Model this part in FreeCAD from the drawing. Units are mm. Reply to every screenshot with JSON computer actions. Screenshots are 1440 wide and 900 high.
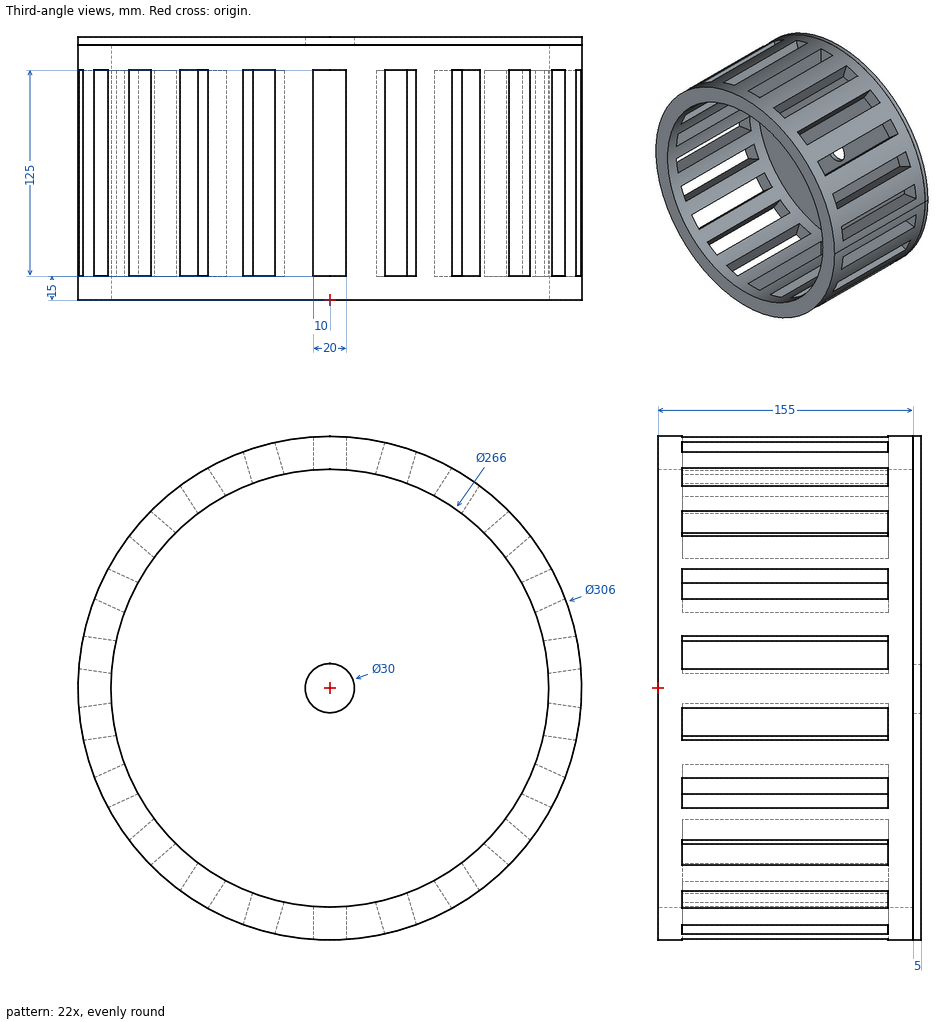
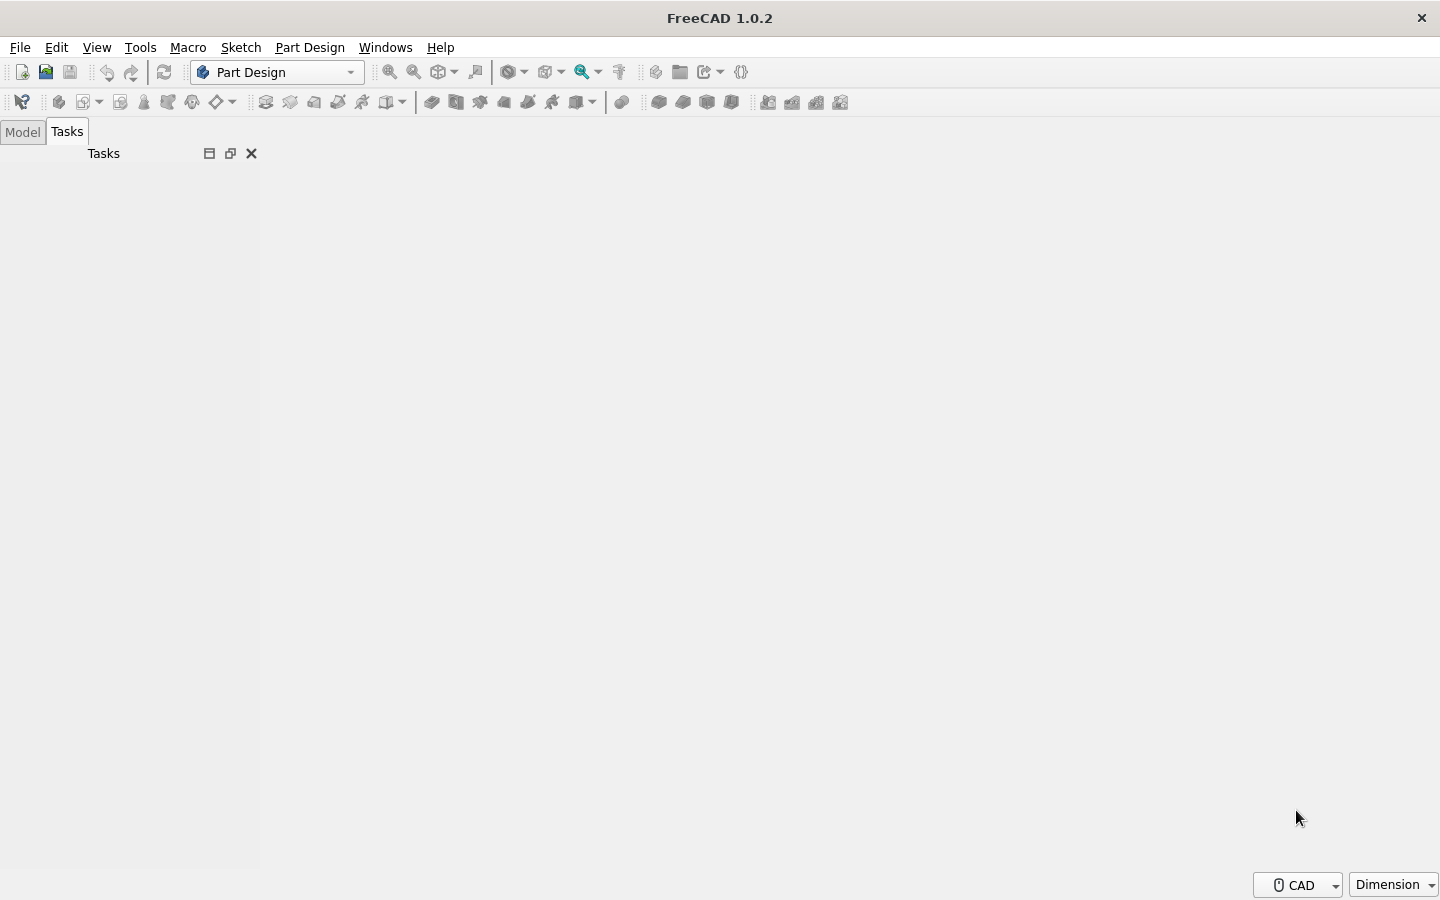
{"action": "left_click", "coordinate": [22, 72]}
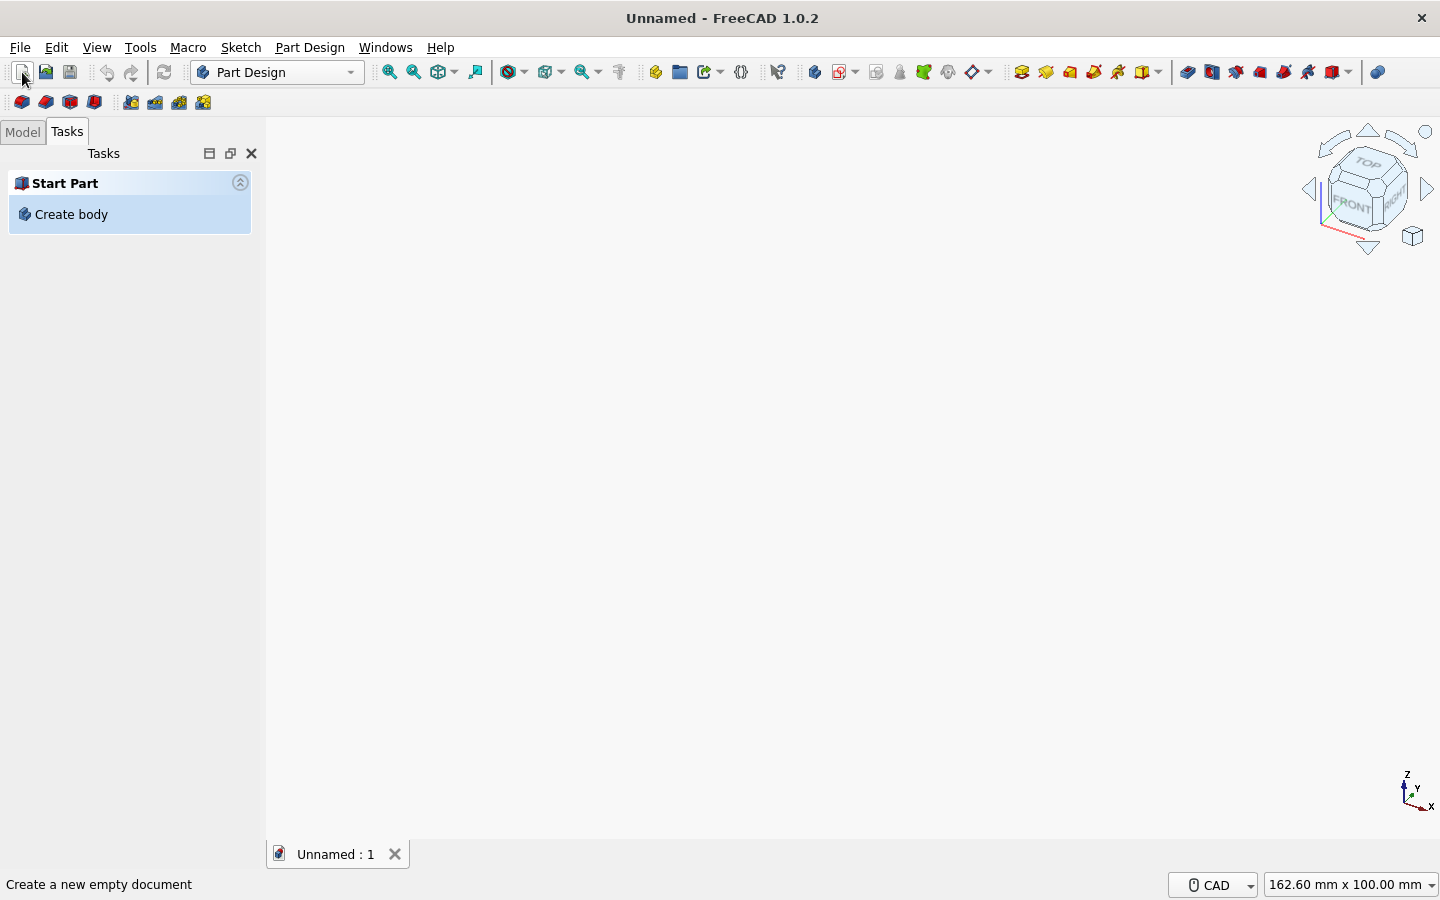
{"action": "left_click", "coordinate": [840, 72]}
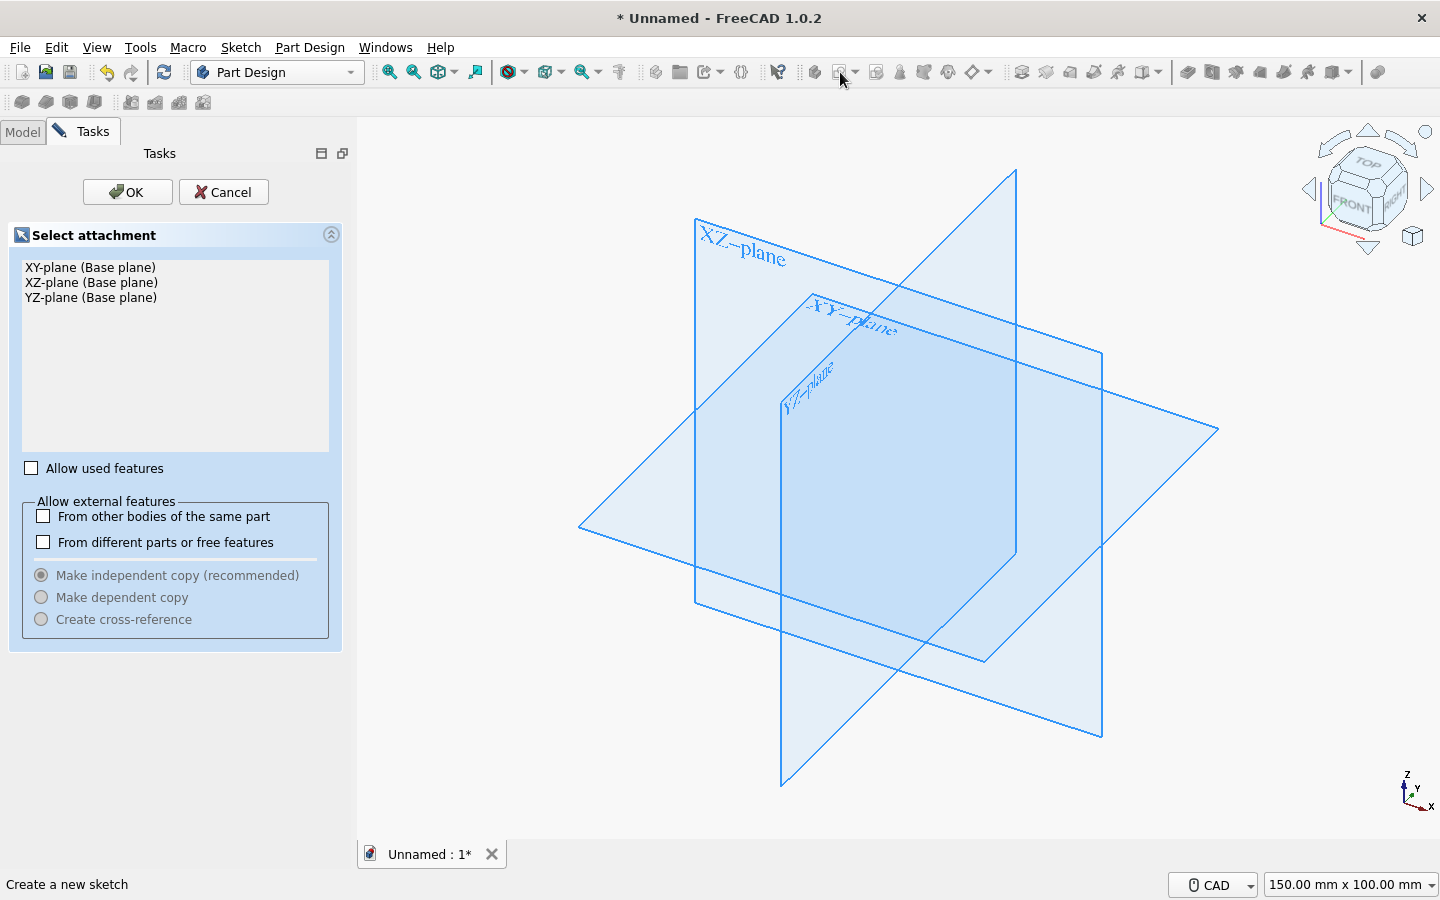
{"action": "left_click", "coordinate": [82, 282]}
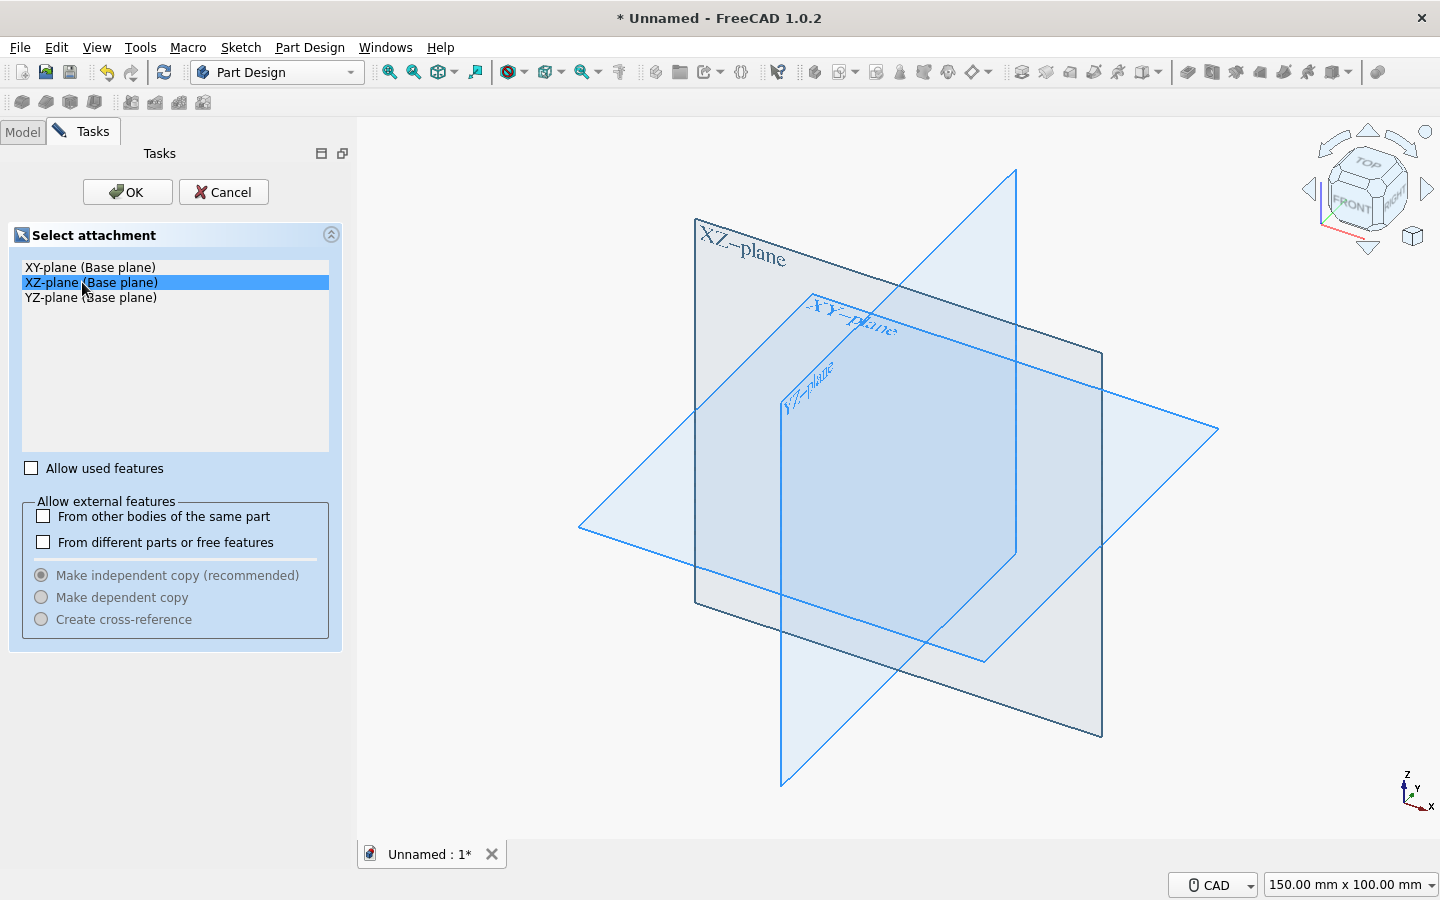
{"action": "left_click", "coordinate": [128, 192]}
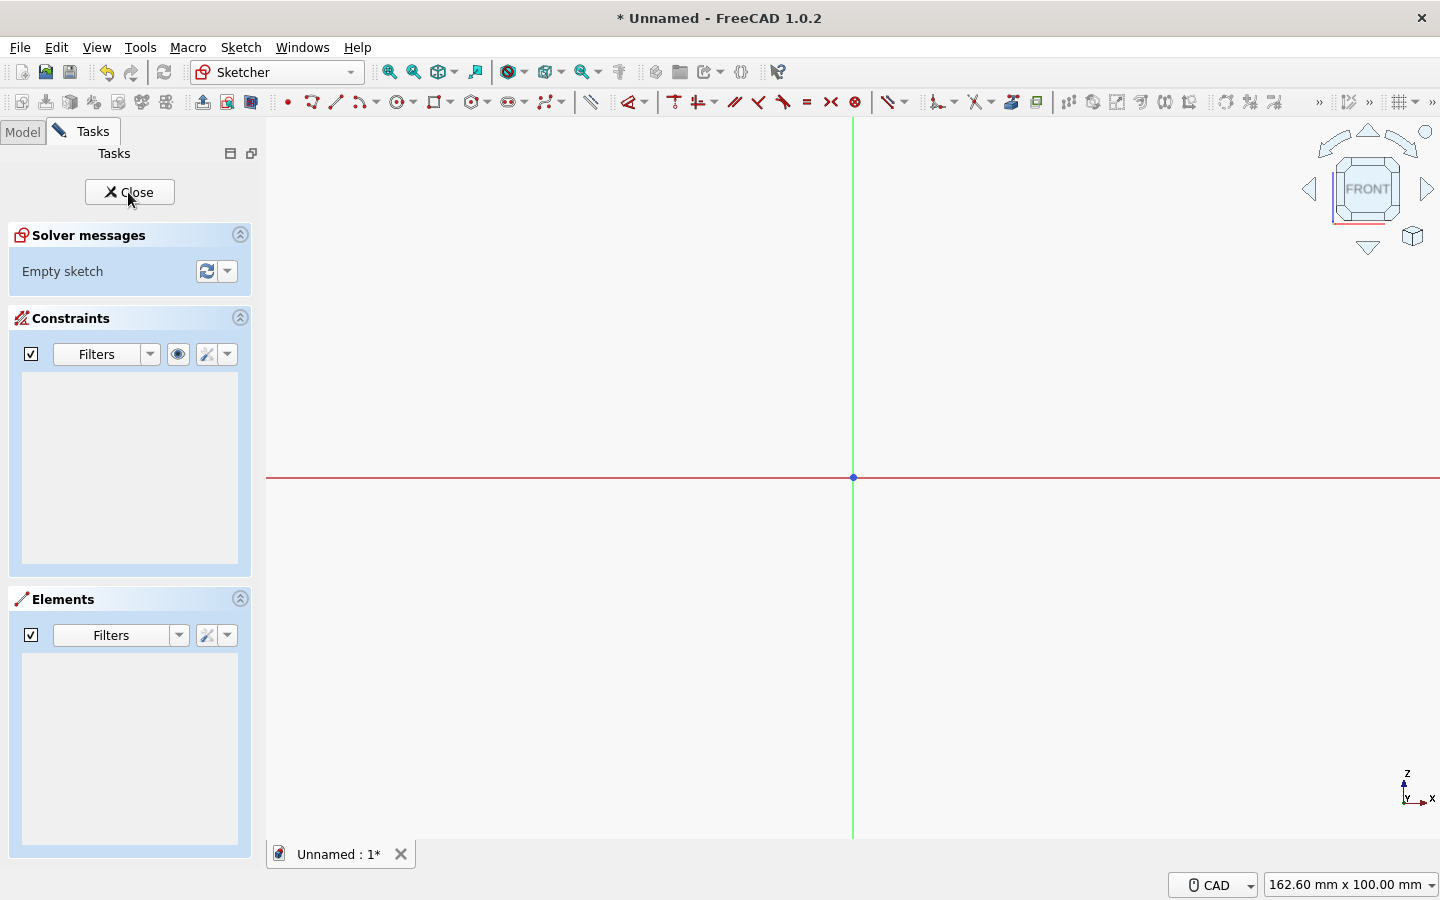
{"action": "scroll", "coordinate": [767, 478], "scroll_direction": "down", "scroll_amount": 8}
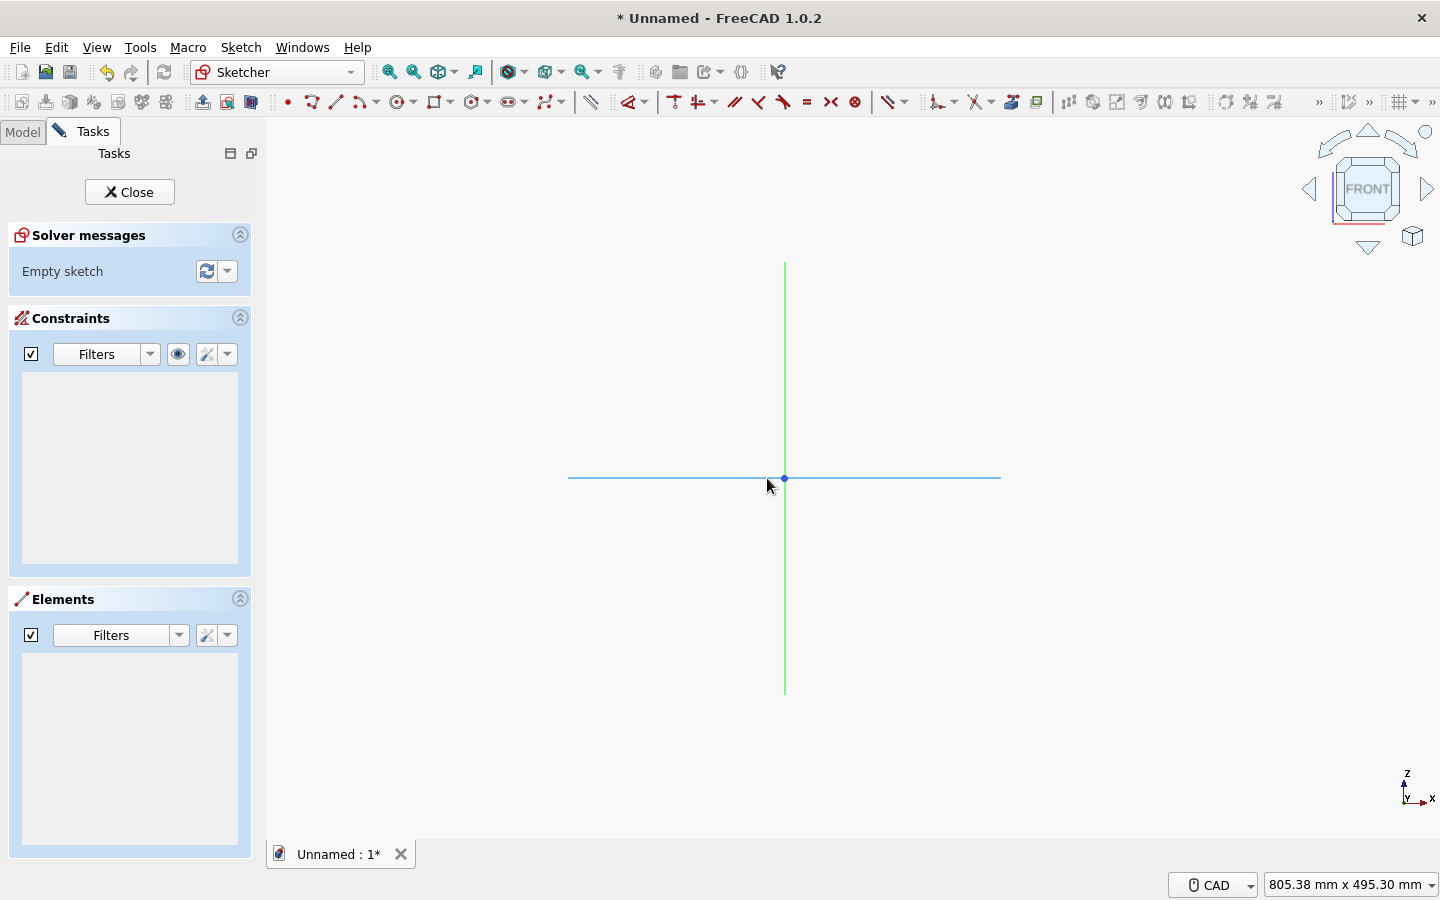
{"action": "left_click", "coordinate": [398, 102]}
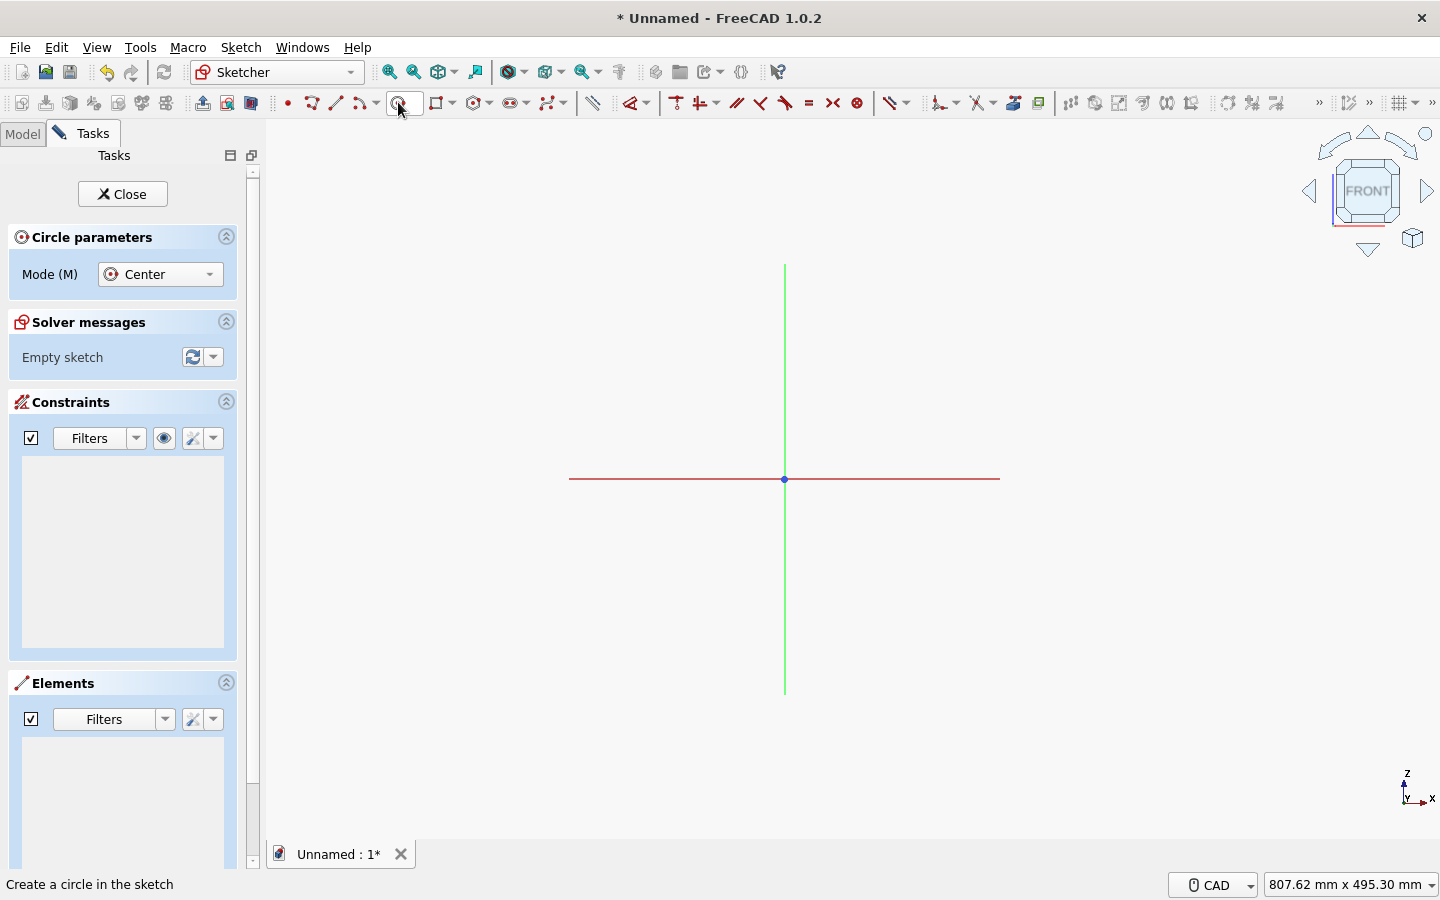
{"action": "left_click", "coordinate": [785, 479]}
{"action": "left_click", "coordinate": [942, 322]}